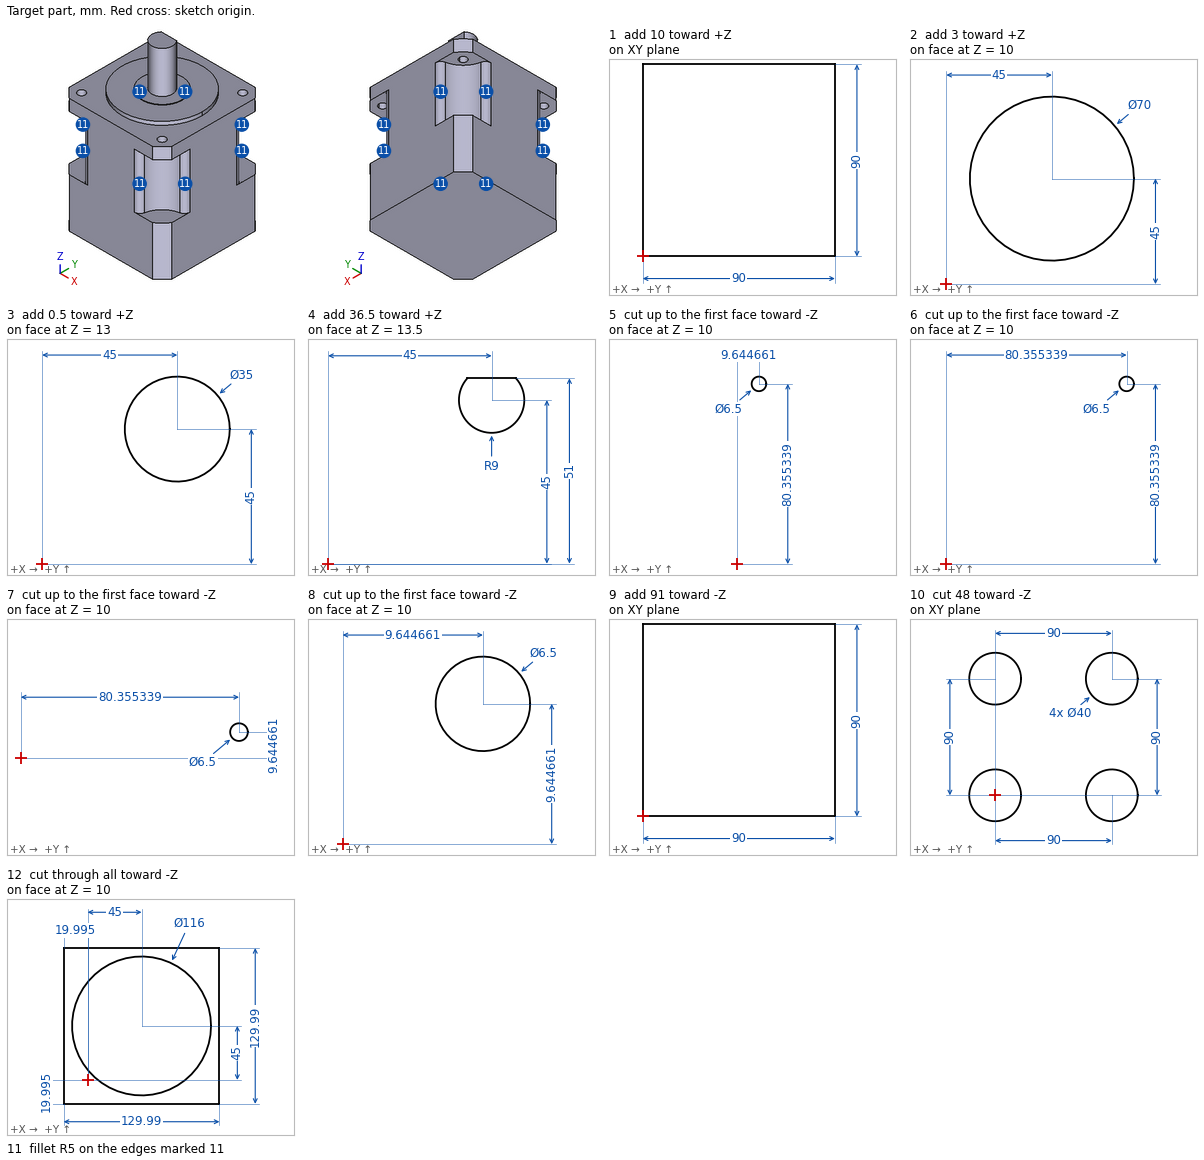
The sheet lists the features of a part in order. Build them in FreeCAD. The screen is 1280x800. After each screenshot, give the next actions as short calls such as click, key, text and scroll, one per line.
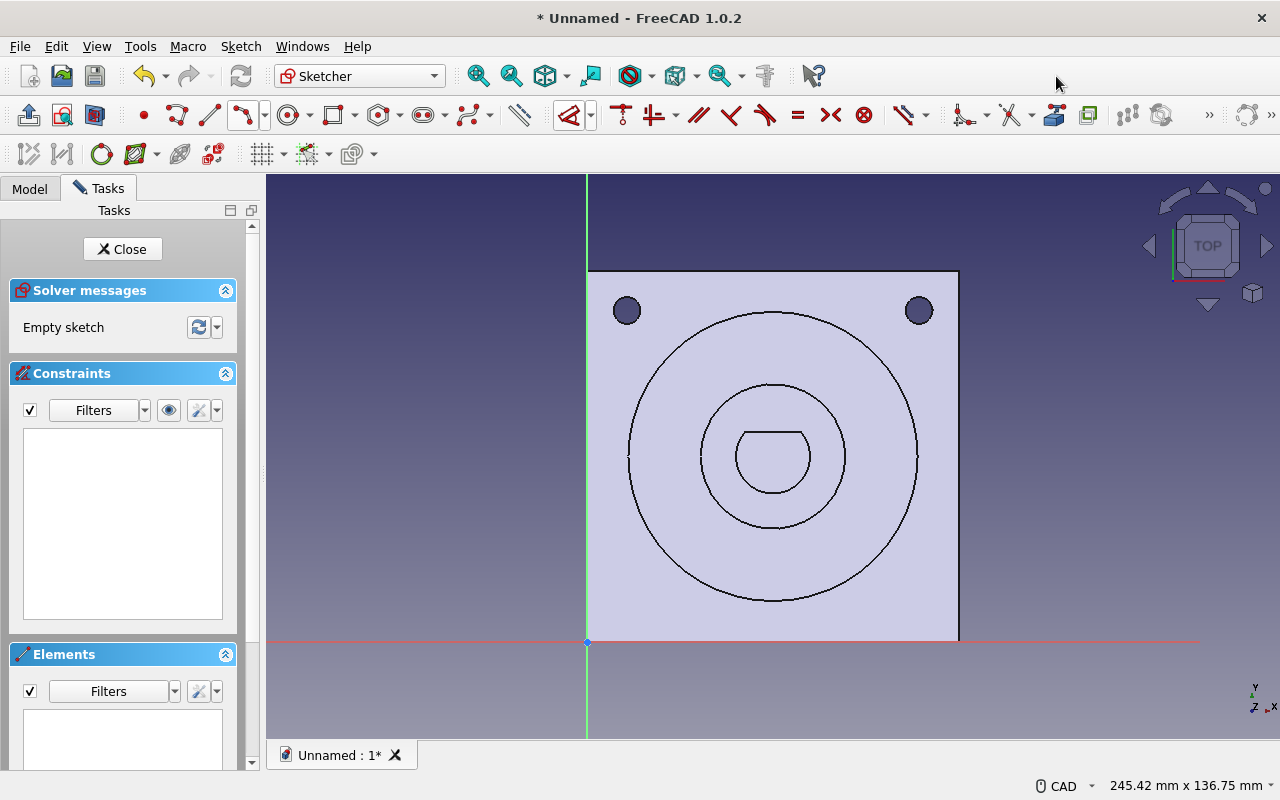
scroll(936, 614, up, 13)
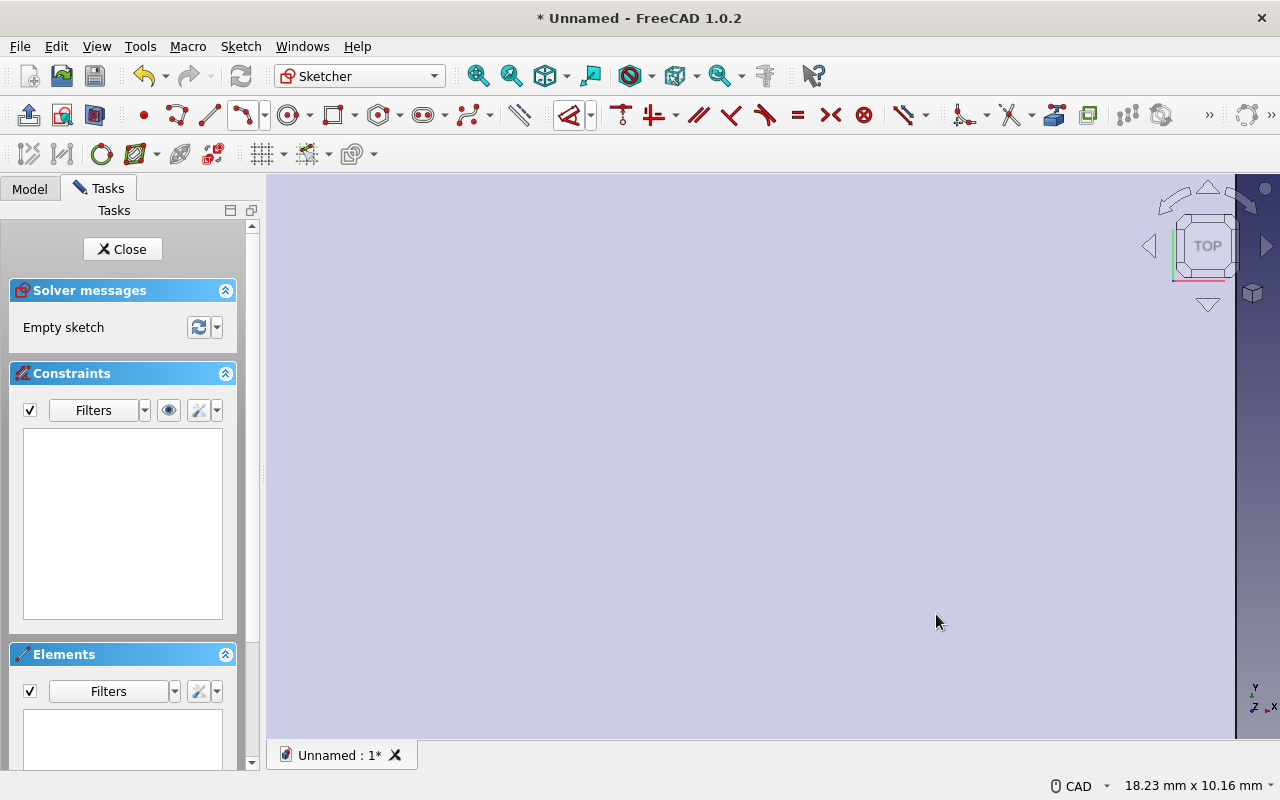
click(288, 116)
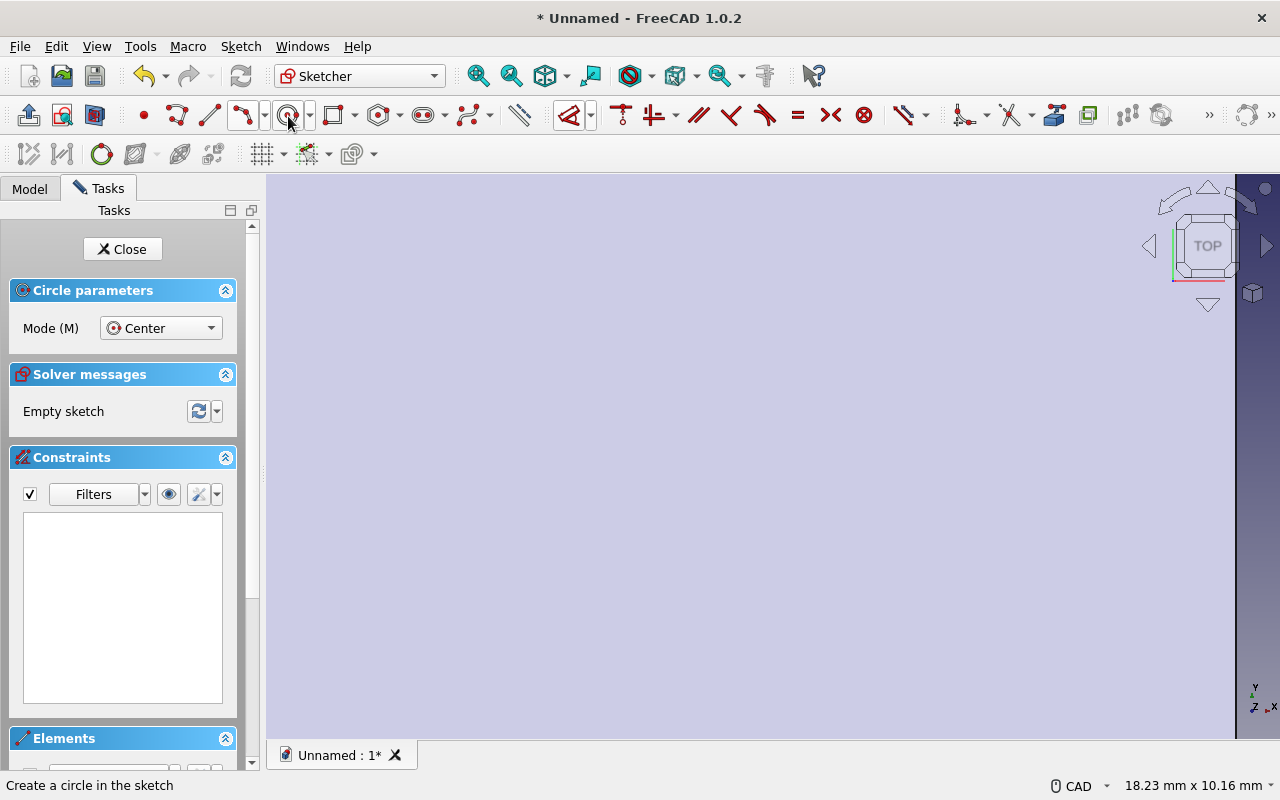
click(700, 450)
move(828, 323)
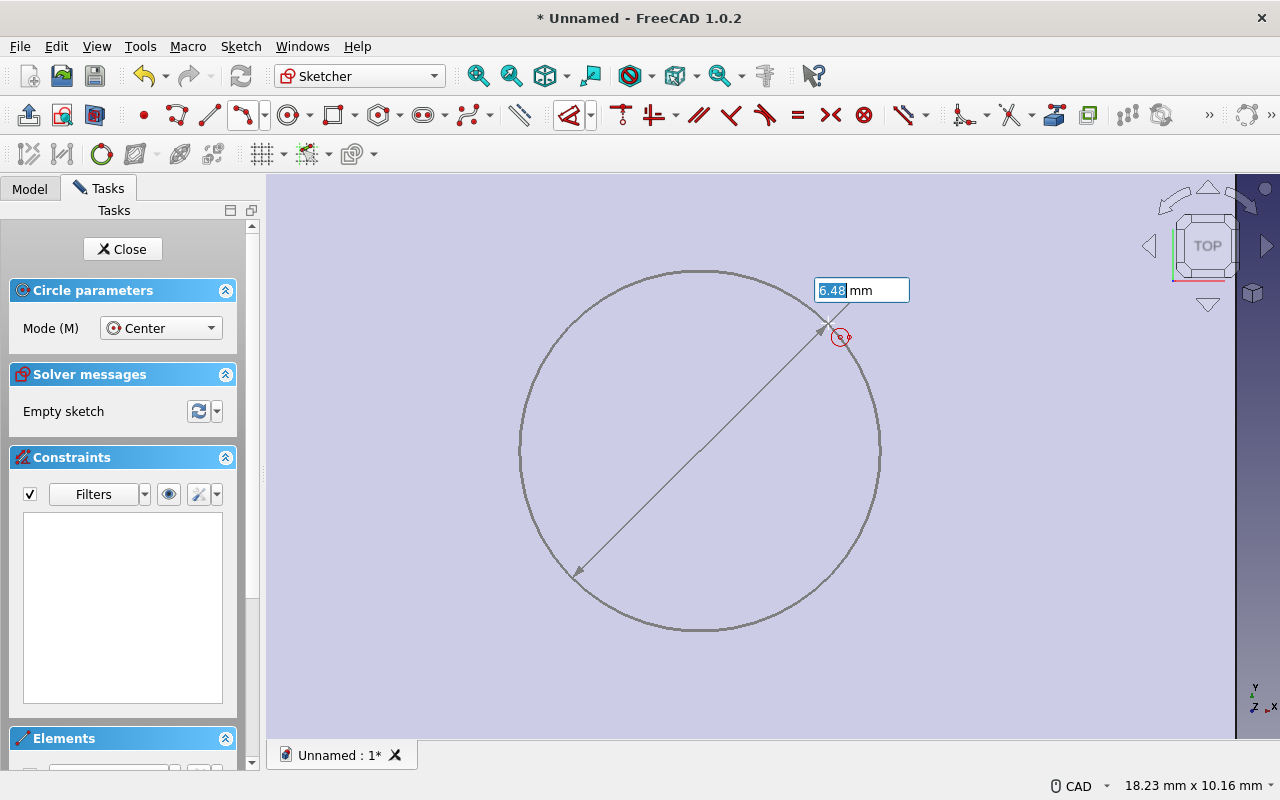
text(6.5)
key(Return)
key(Escape)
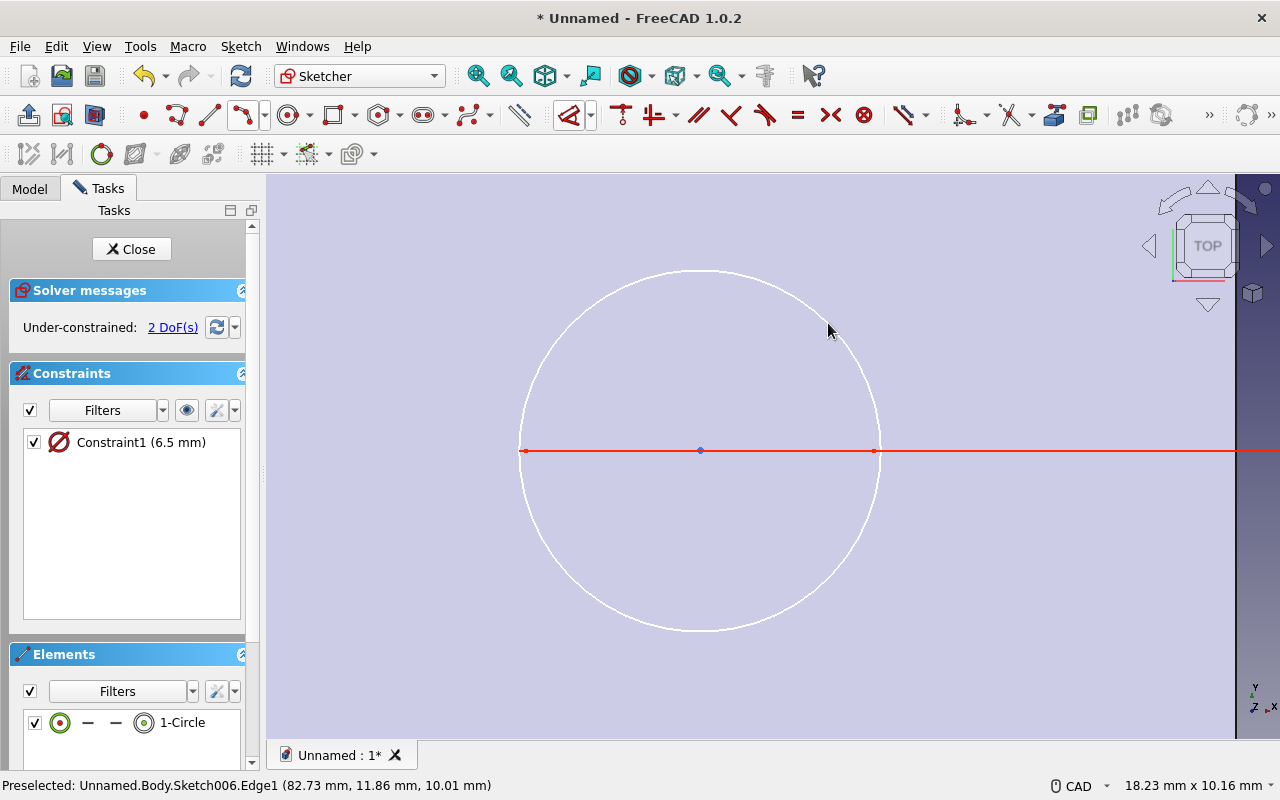
click(700, 451)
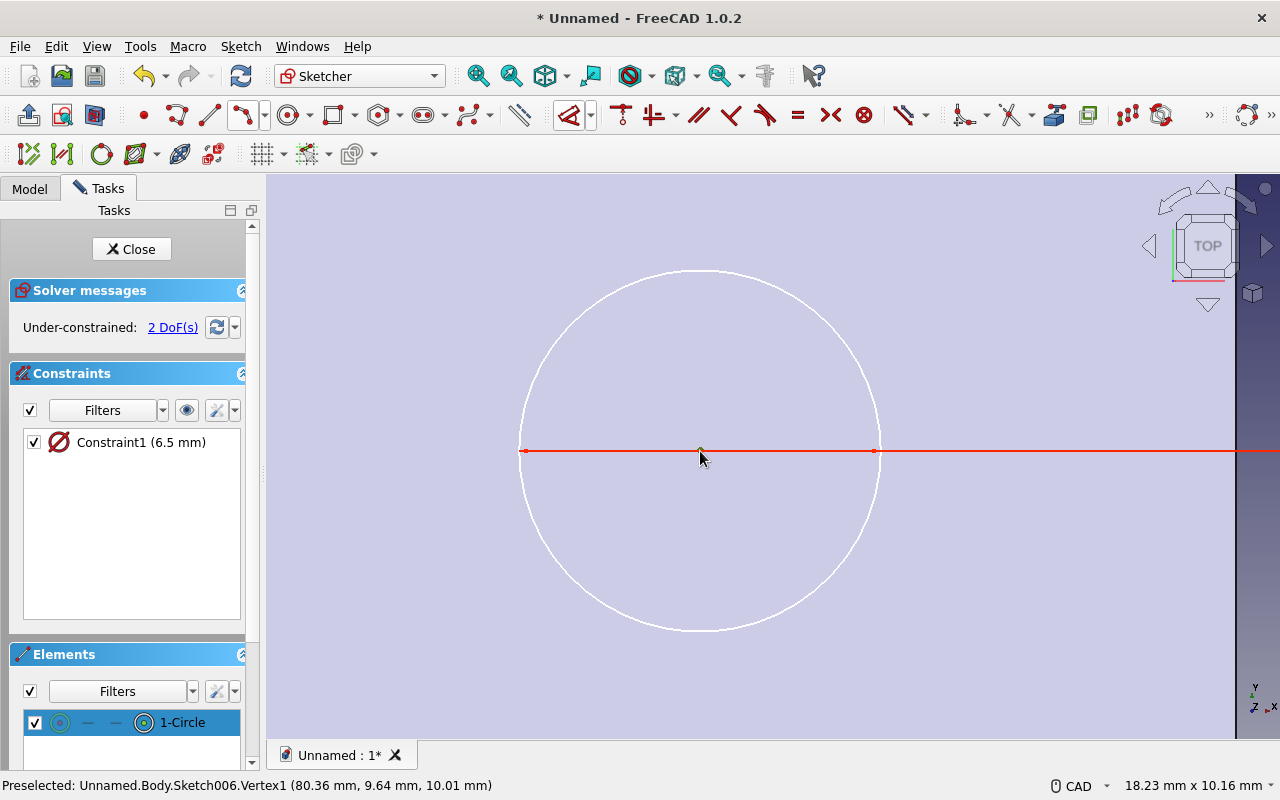
key(i)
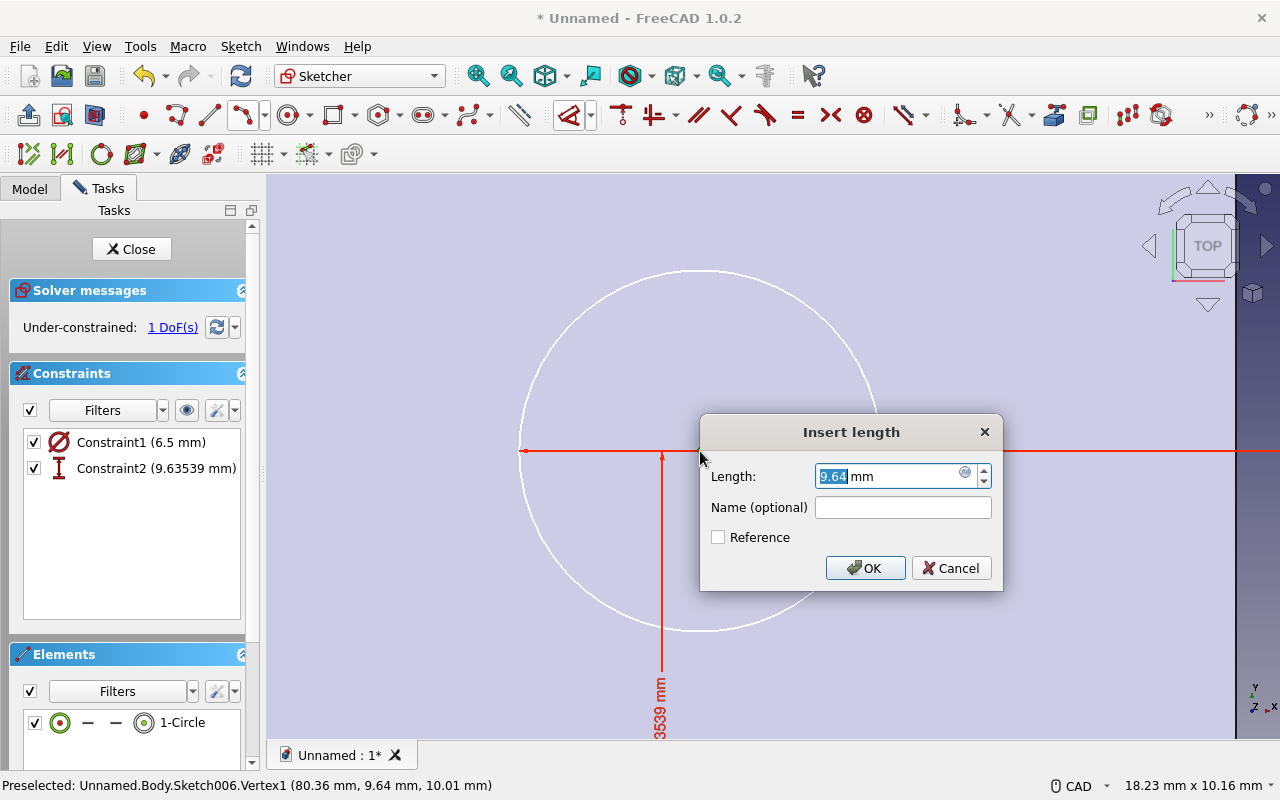
text(9.644661)
key(Return)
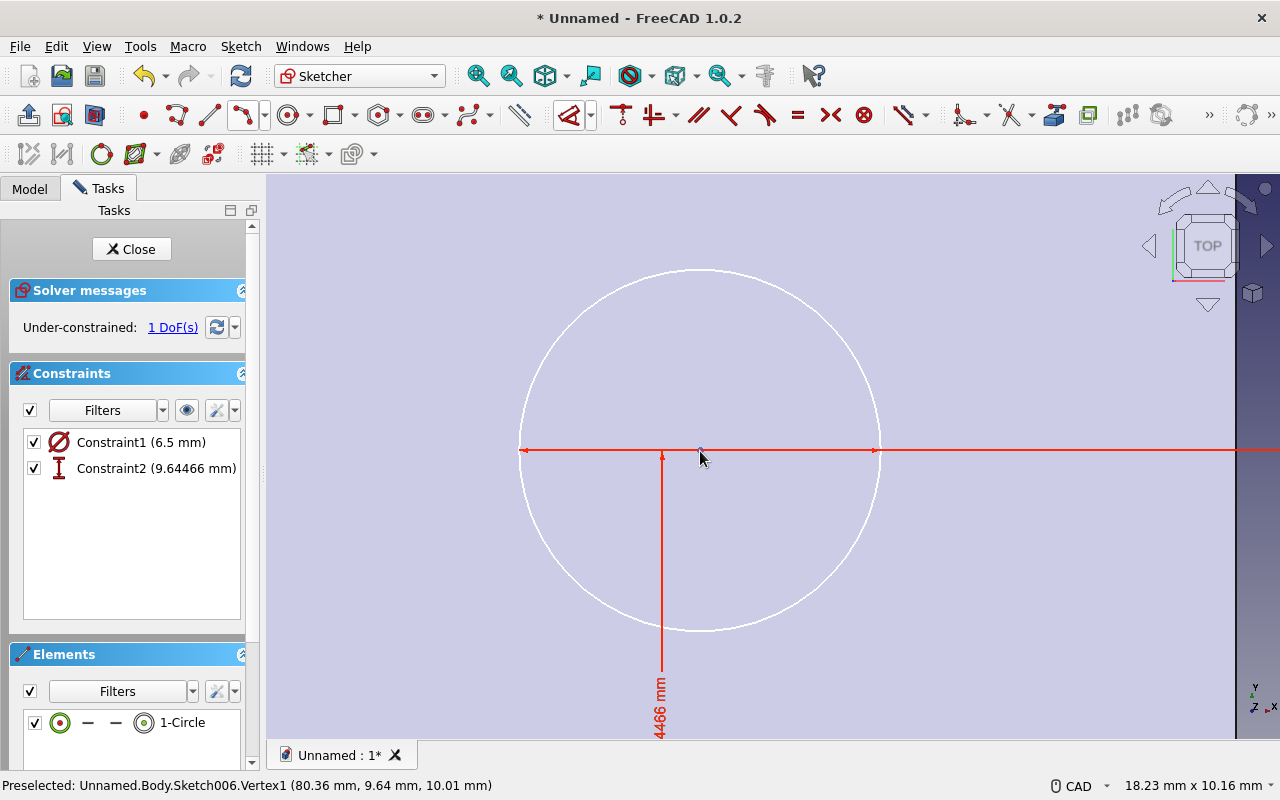
click(700, 450)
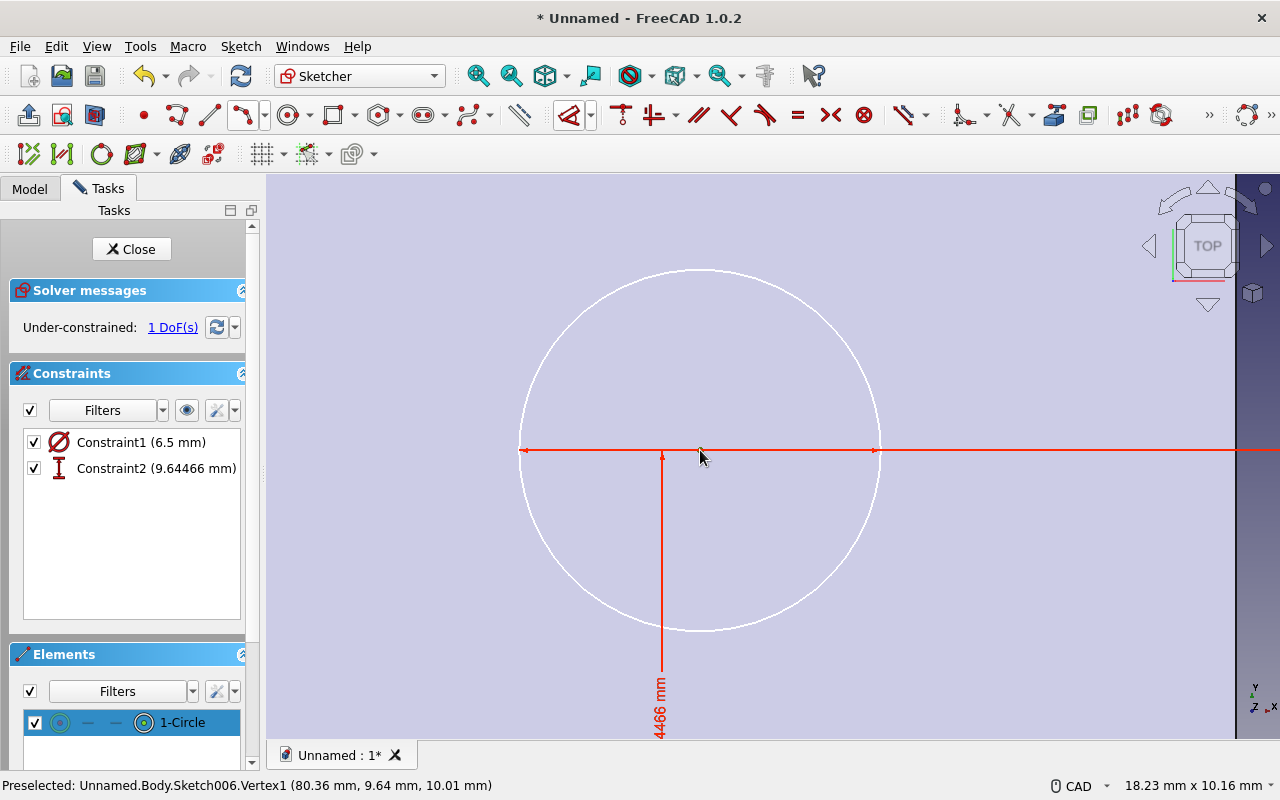
key(l)